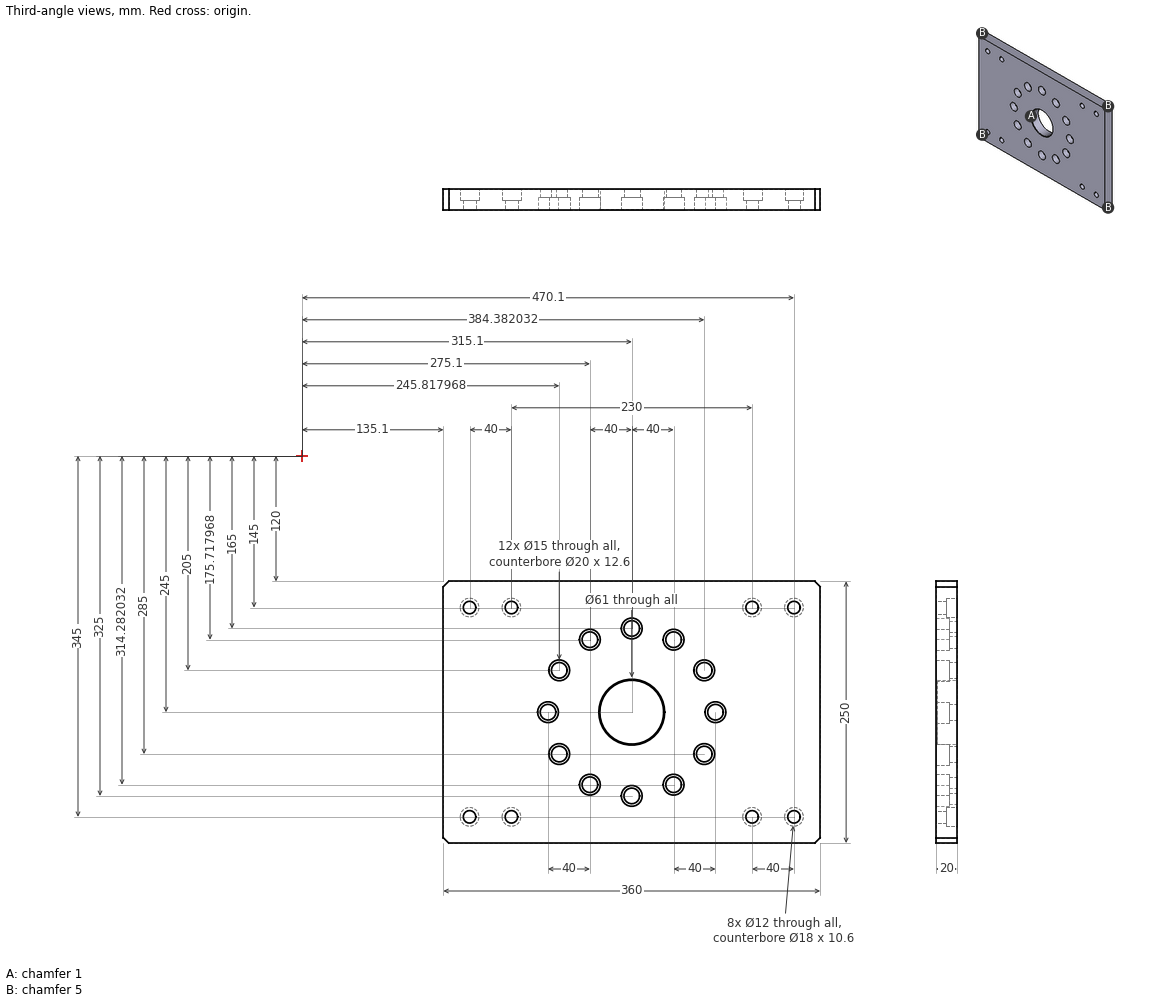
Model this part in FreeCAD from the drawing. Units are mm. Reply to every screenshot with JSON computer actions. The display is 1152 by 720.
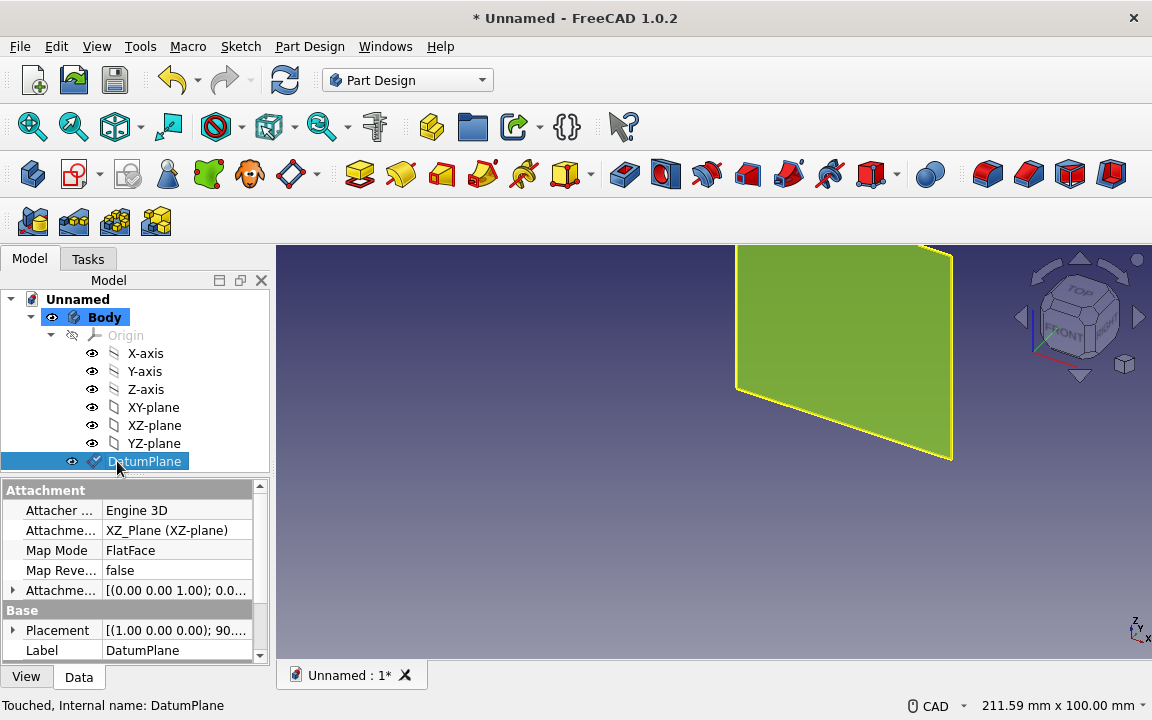
{"action": "left_click", "coordinate": [74, 174]}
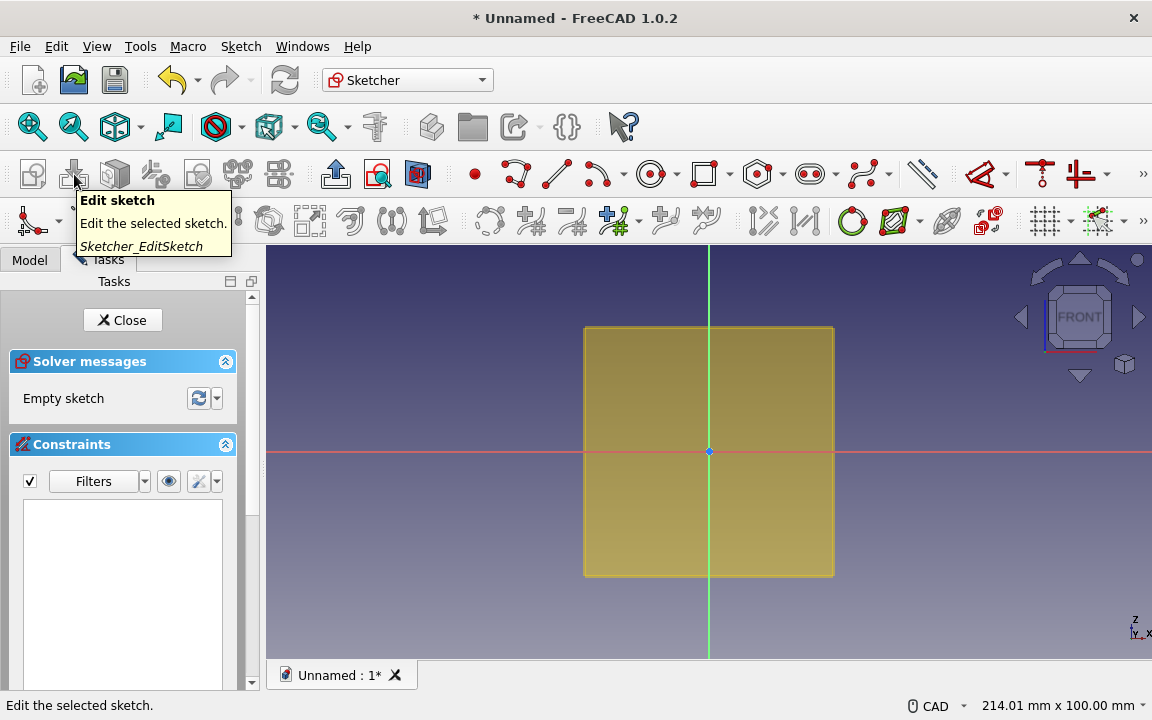
{"action": "scroll", "coordinate": [424, 300], "scroll_direction": "down", "scroll_amount": 9}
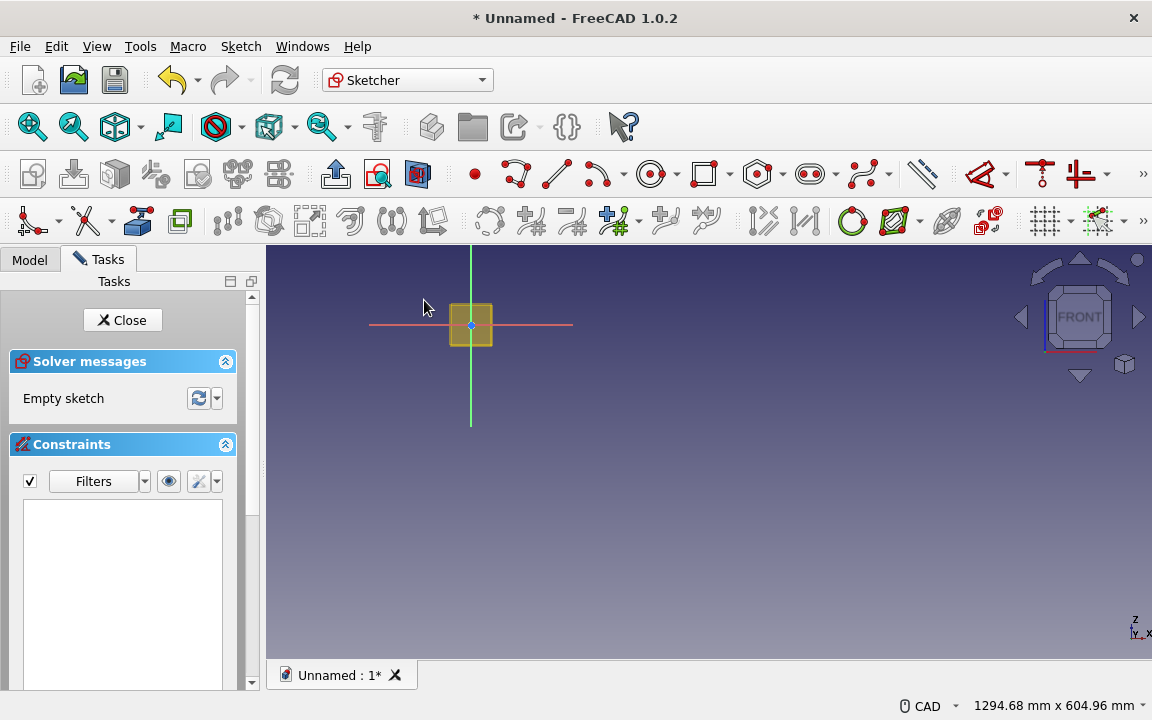
{"action": "left_click", "coordinate": [704, 174]}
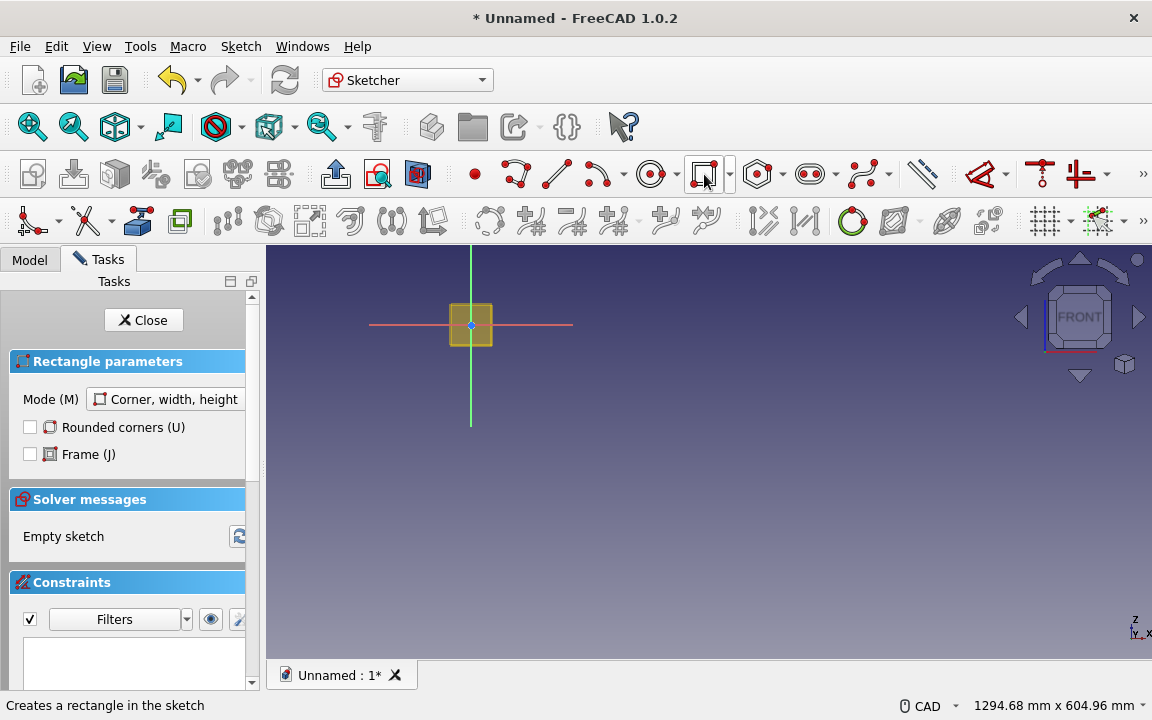
{"action": "left_click", "coordinate": [564, 407]}
{"action": "mouse_move", "coordinate": [810, 578]}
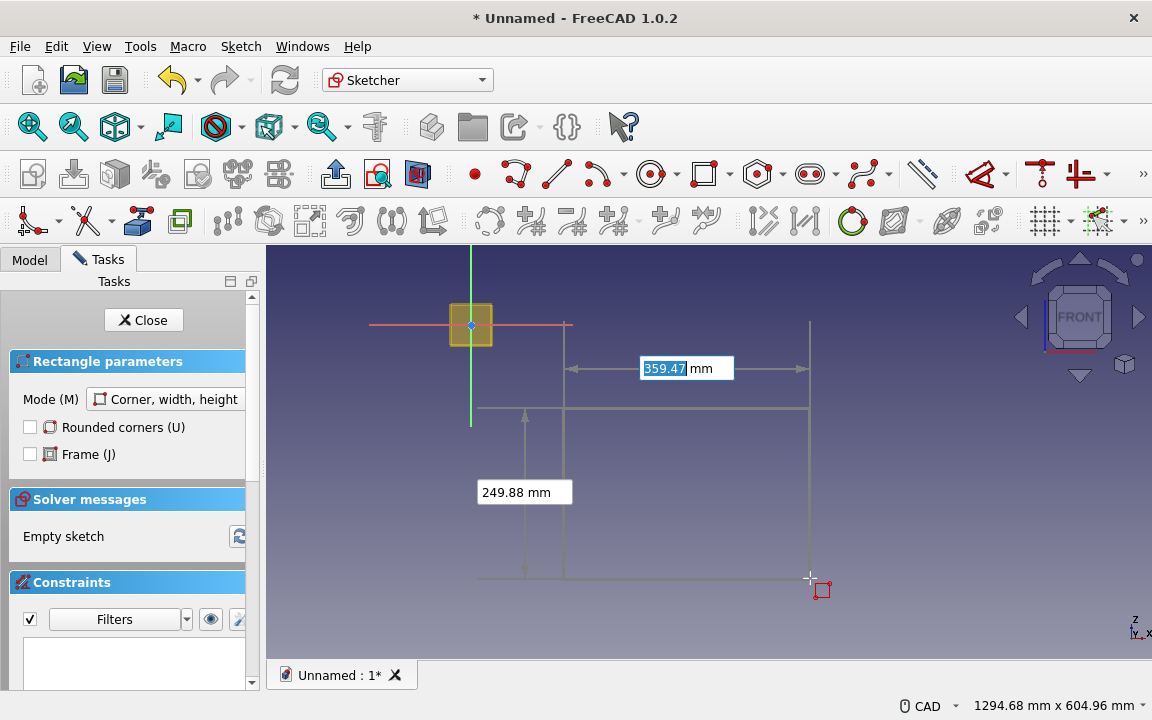
{"action": "type", "text": "360"}
{"action": "key", "text": "Tab"}
{"action": "type", "text": "250"}
{"action": "key", "text": "Return"}
{"action": "key", "text": "Escape"}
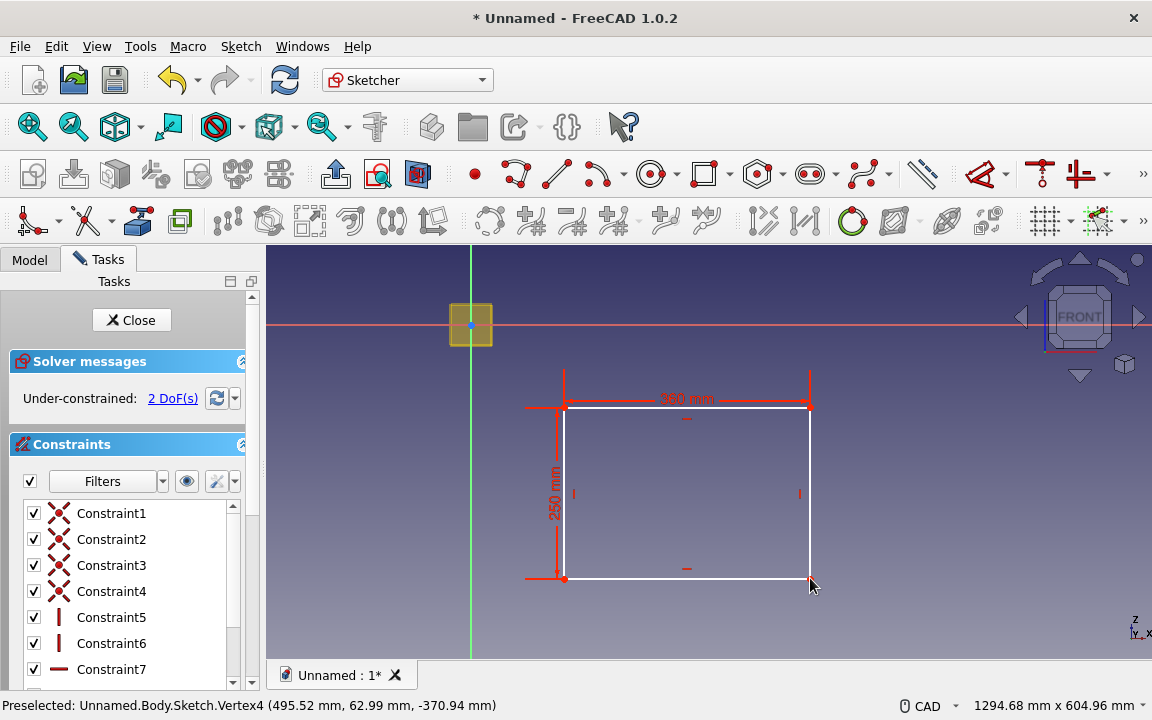
{"action": "left_click", "coordinate": [980, 174]}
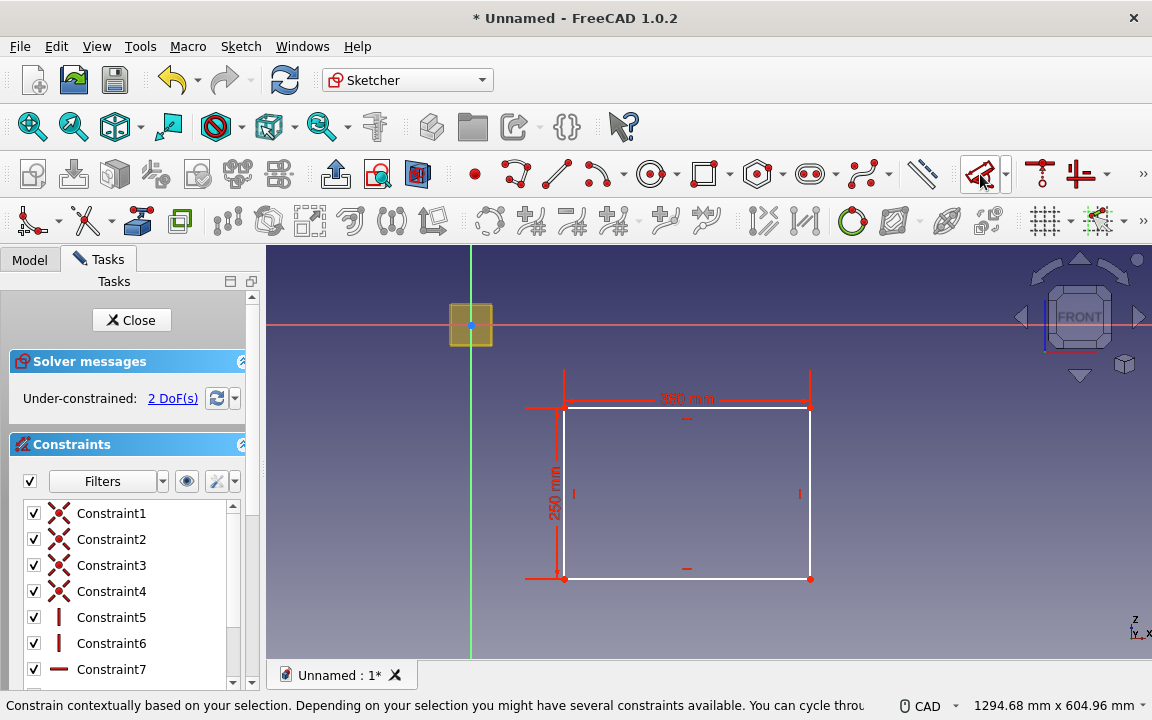
{"action": "left_click", "coordinate": [564, 408]}
{"action": "left_click", "coordinate": [437, 367]}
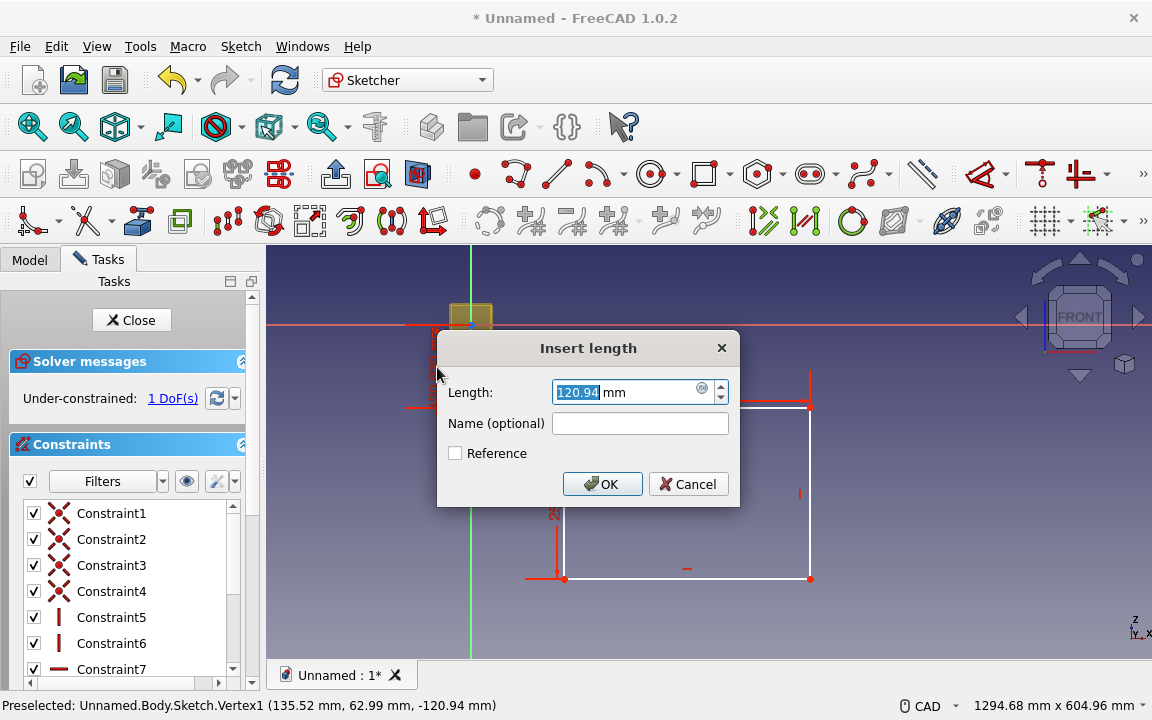
{"action": "type", "text": "120"}
{"action": "key", "text": "Return"}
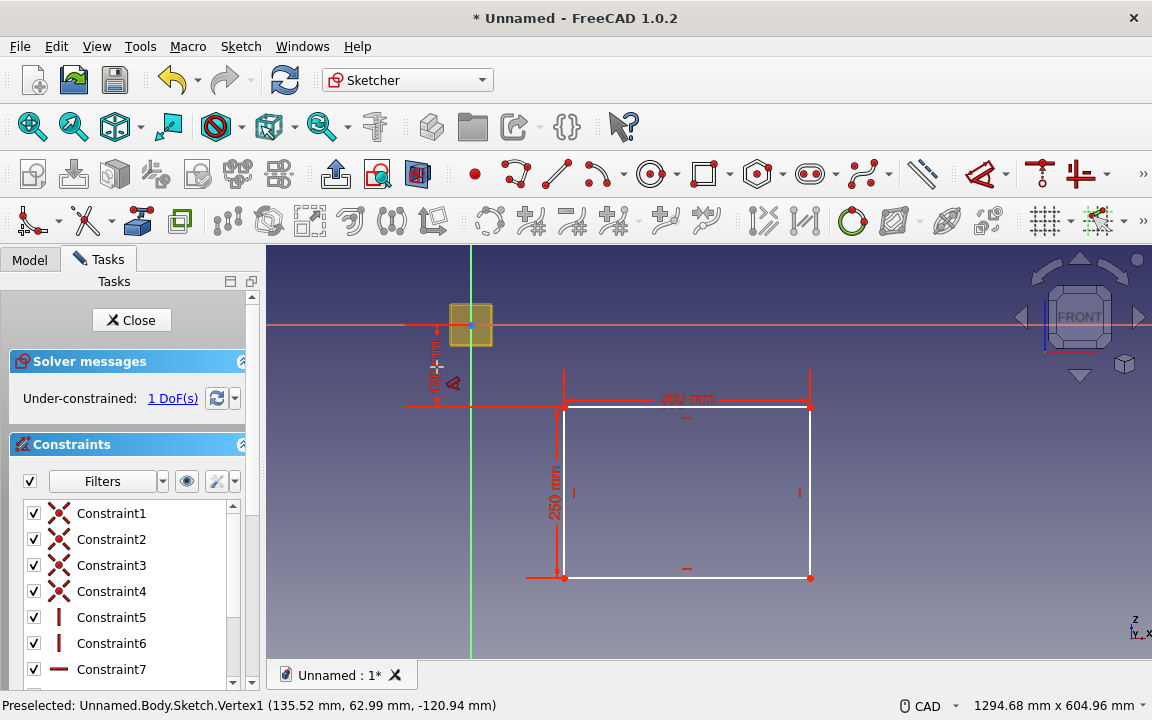
{"action": "left_click", "coordinate": [564, 407]}
{"action": "left_click", "coordinate": [518, 291]}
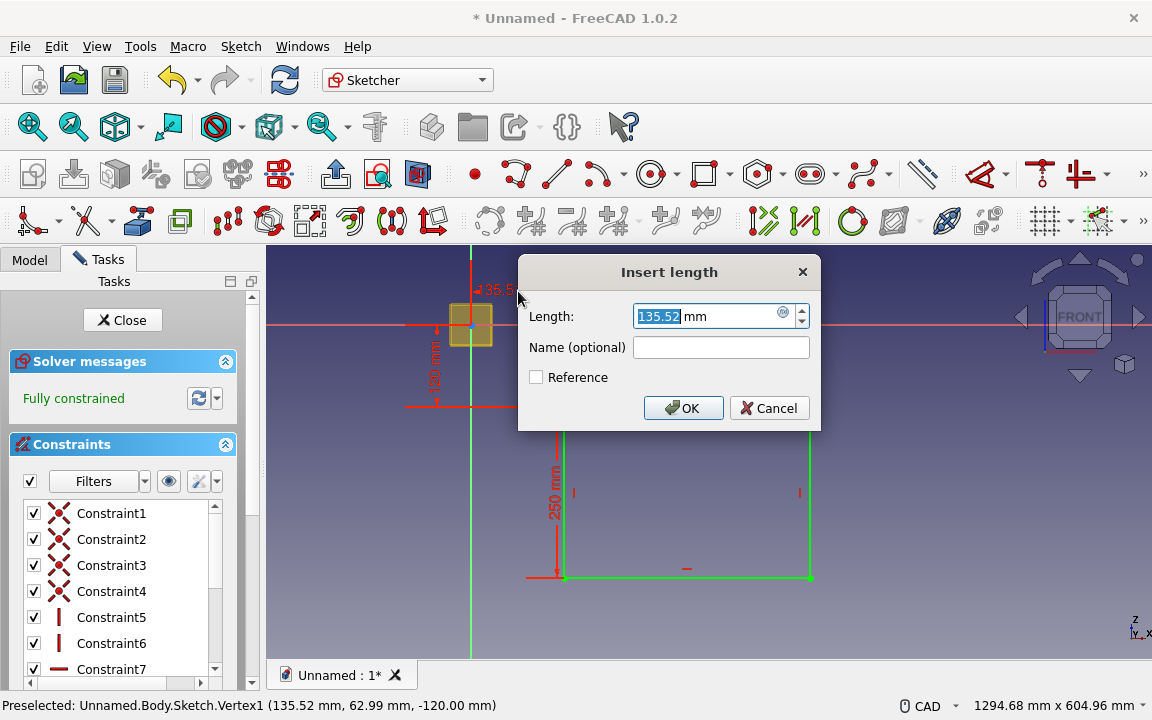
{"action": "type", "text": "135.1"}
{"action": "key", "text": "Return"}
{"action": "key", "text": "Escape"}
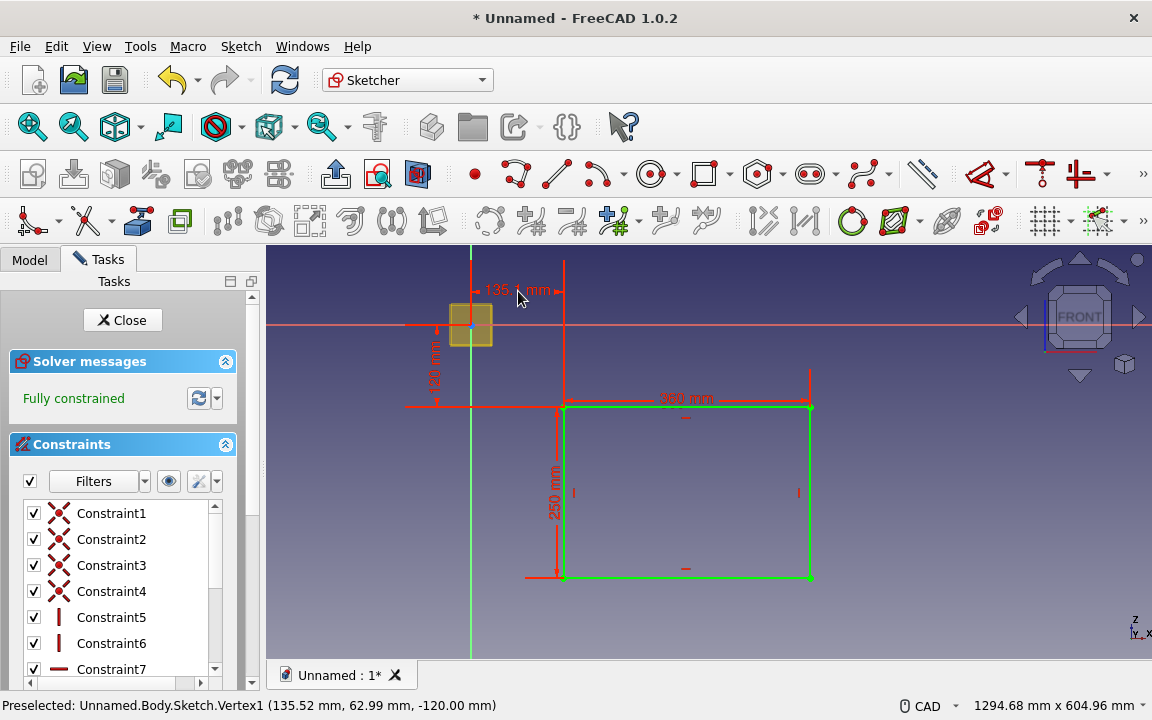
{"action": "left_click", "coordinate": [123, 320]}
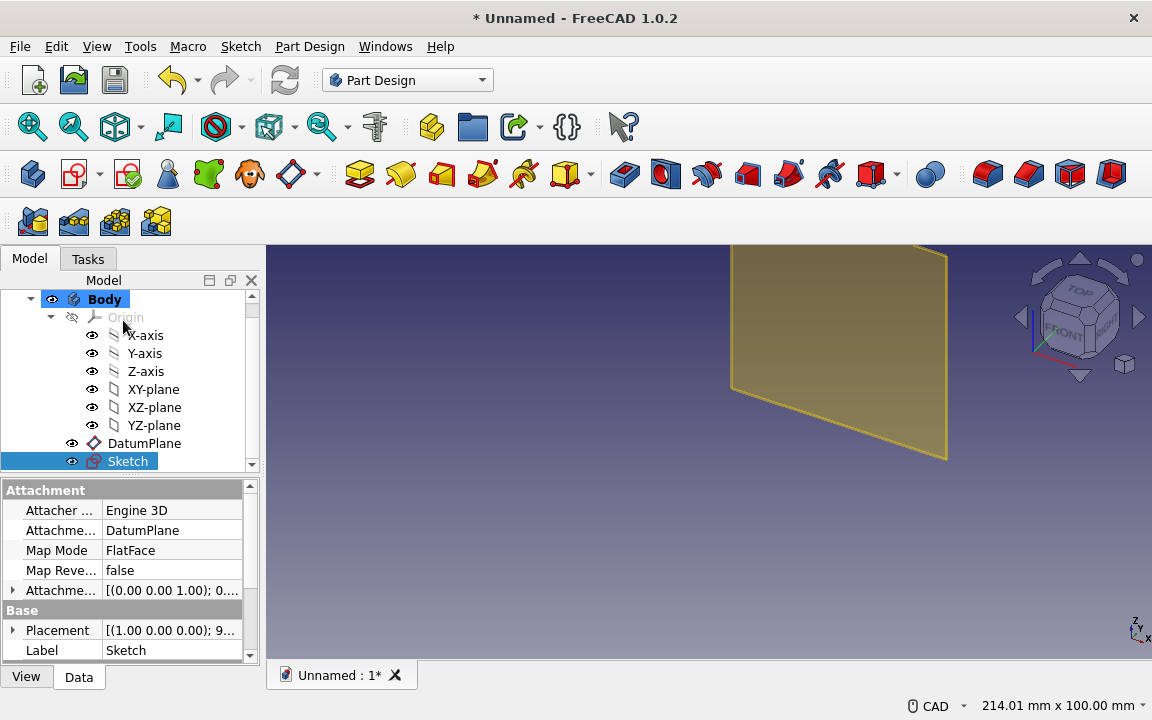
{"action": "left_click", "coordinate": [360, 174]}